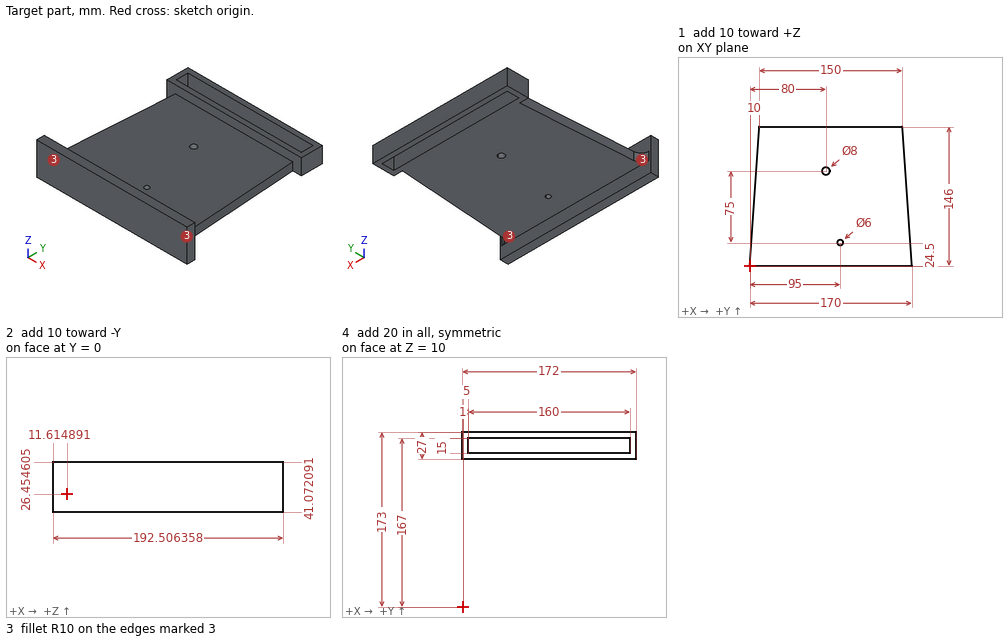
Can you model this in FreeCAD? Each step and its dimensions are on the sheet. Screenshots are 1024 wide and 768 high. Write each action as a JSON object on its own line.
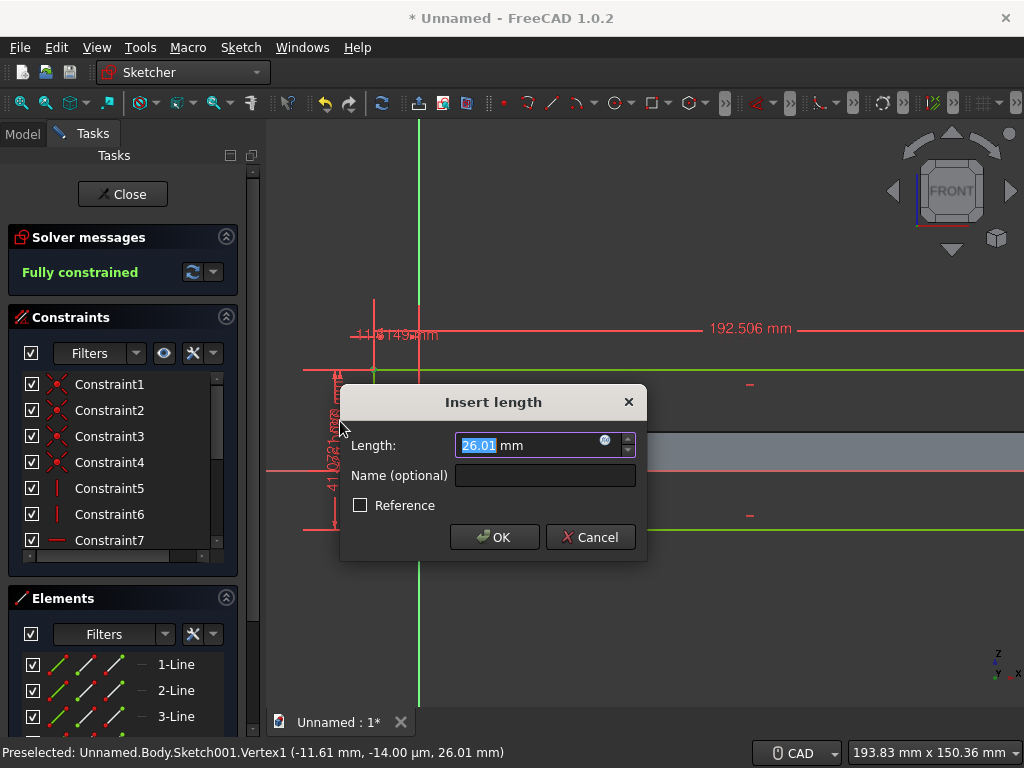
{"action": "type", "text": "26.454605"}
{"action": "key", "text": "Return"}
{"action": "key", "text": "Escape"}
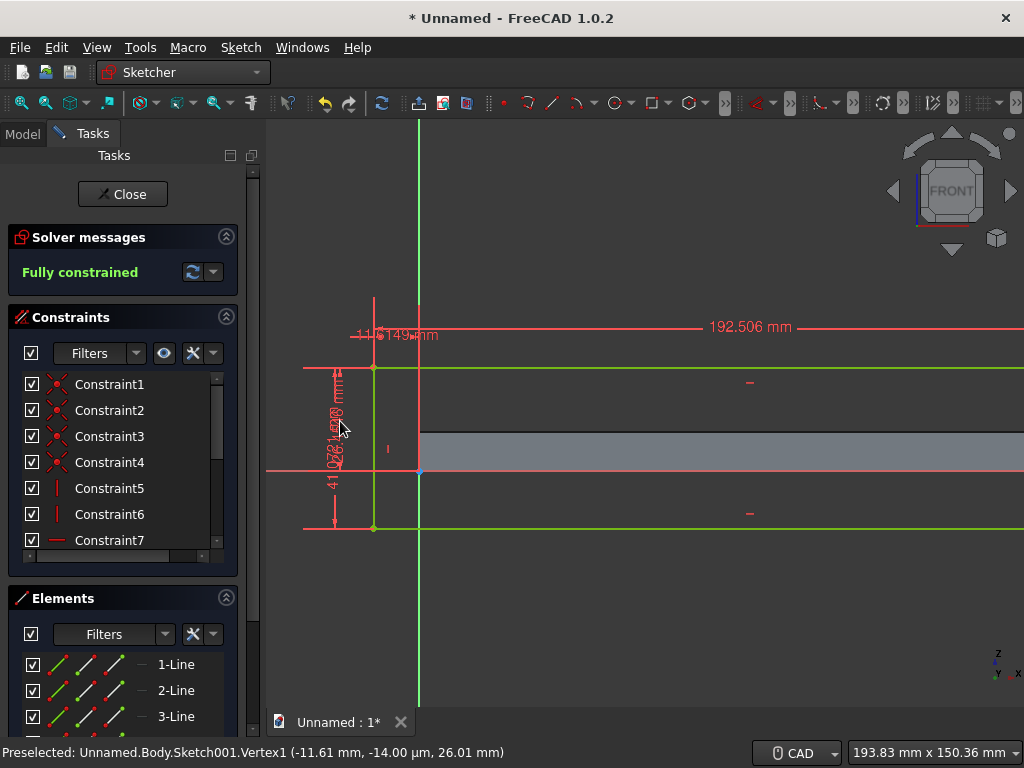
{"action": "left_click", "coordinate": [123, 194]}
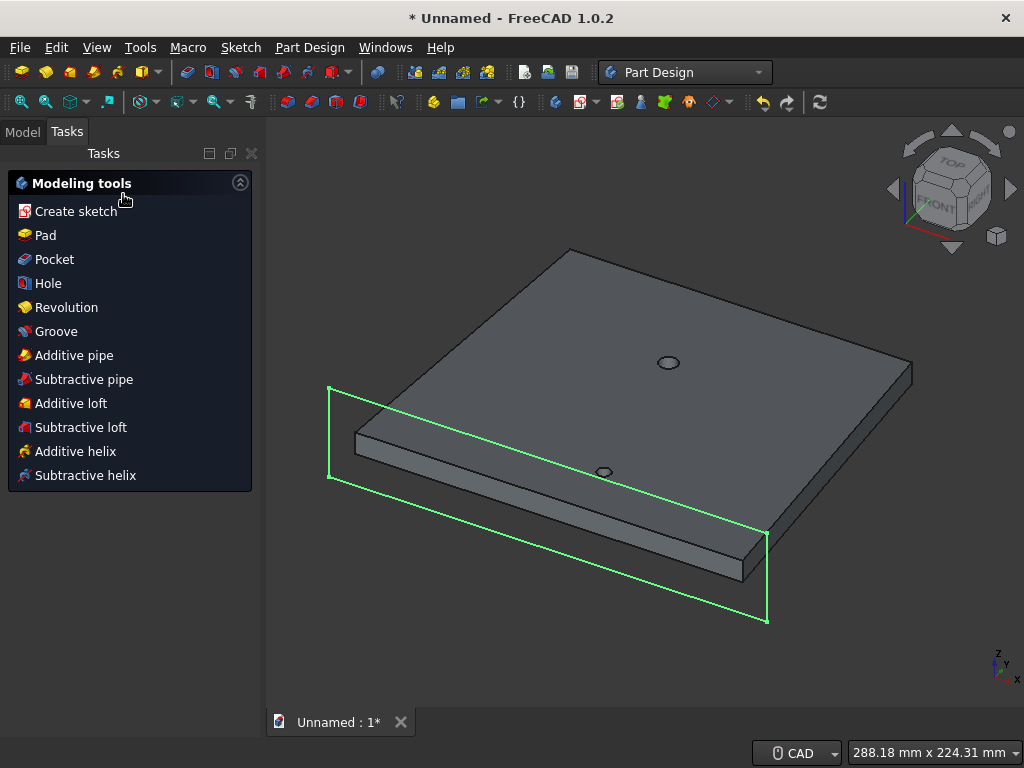
{"action": "left_click", "coordinate": [22, 72]}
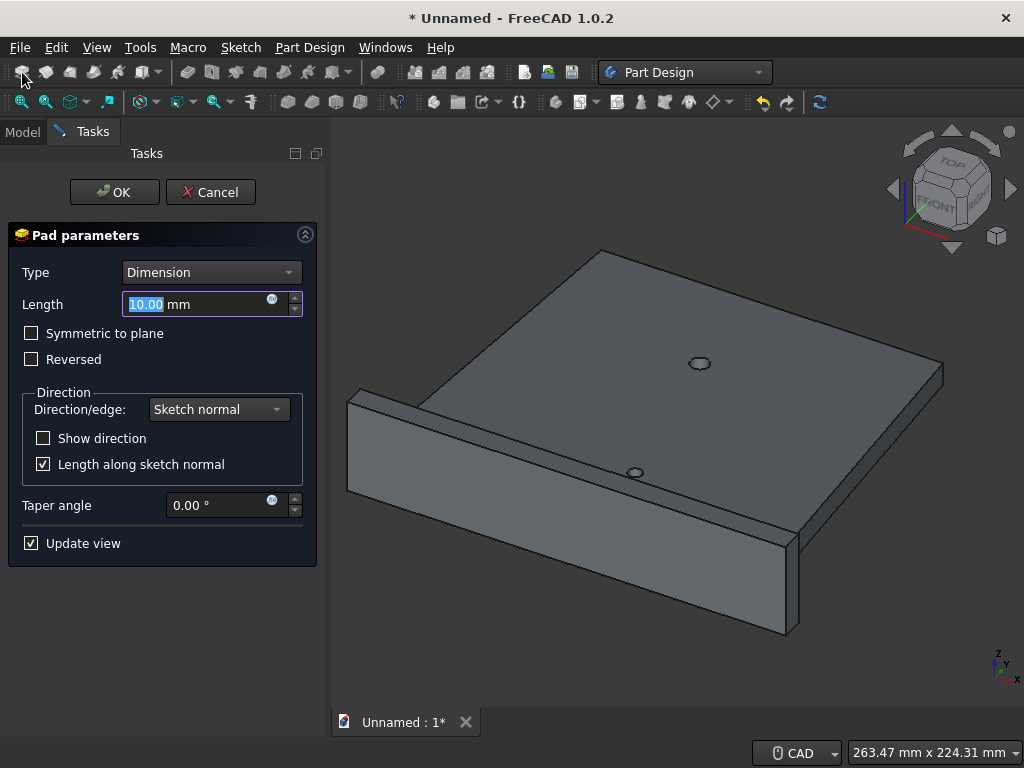
{"action": "type", "text": "10"}
{"action": "key", "text": "Tab"}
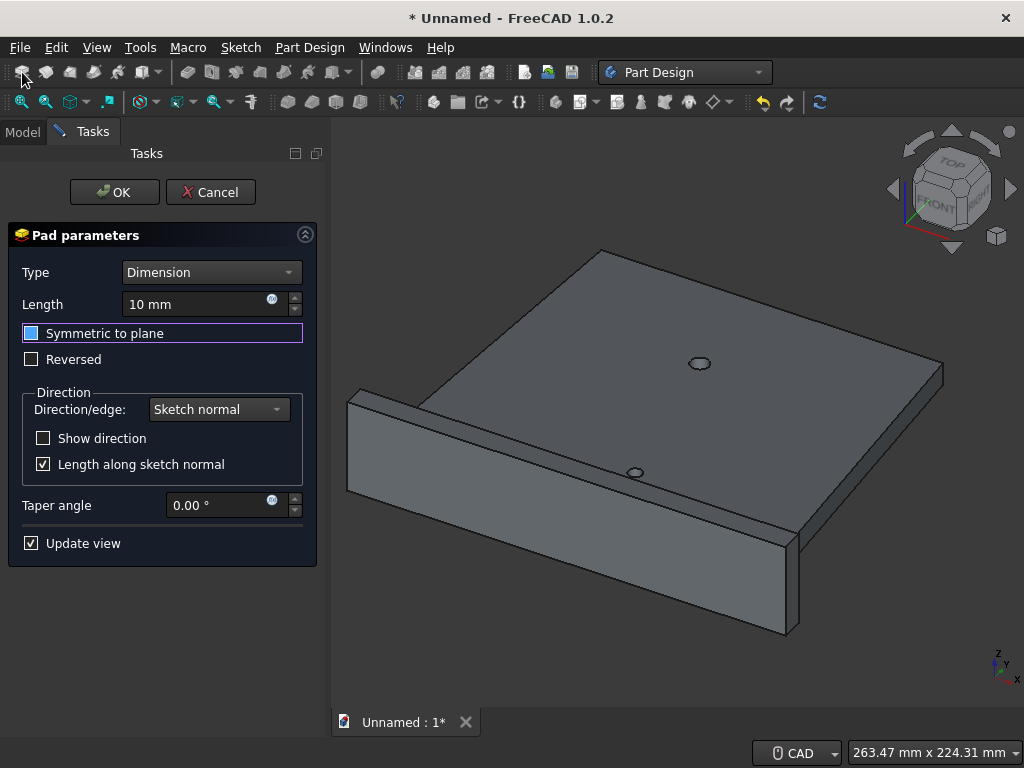
{"action": "left_click", "coordinate": [115, 192]}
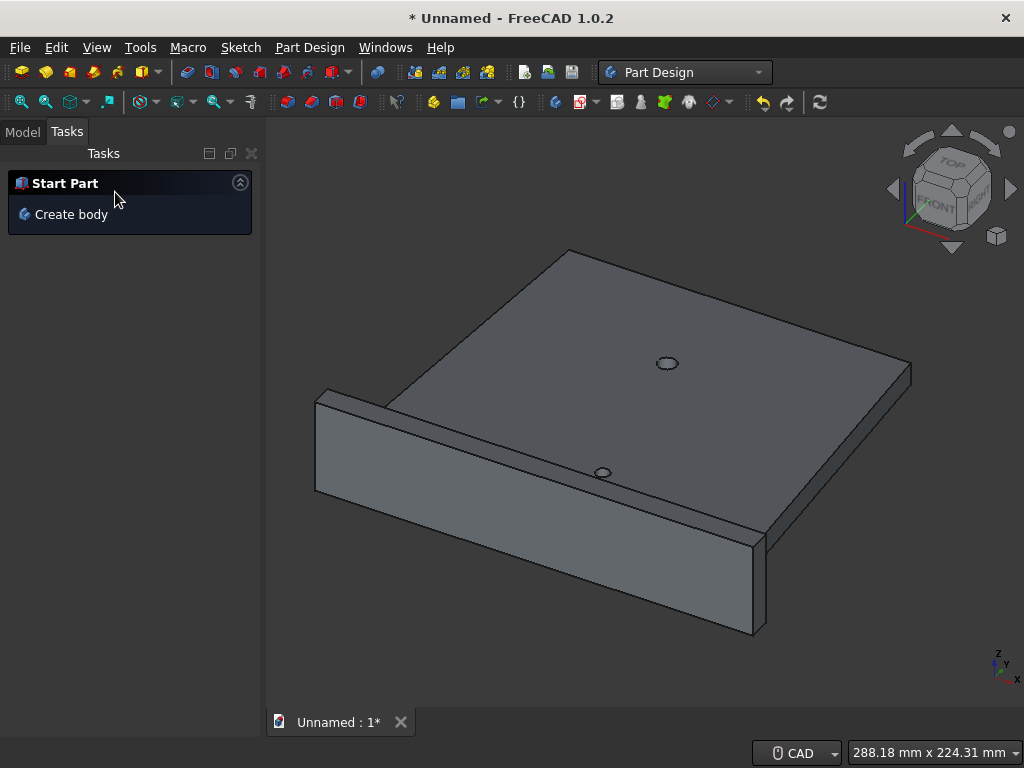
{"action": "key", "text": "0"}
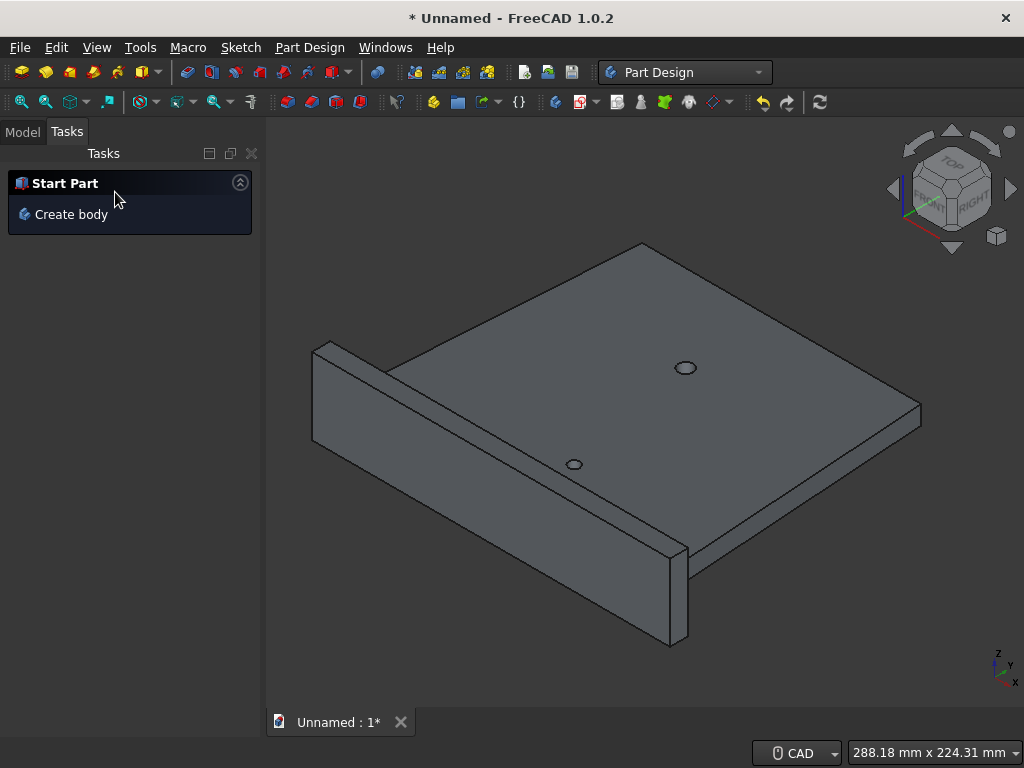
{"action": "key", "text": "2"}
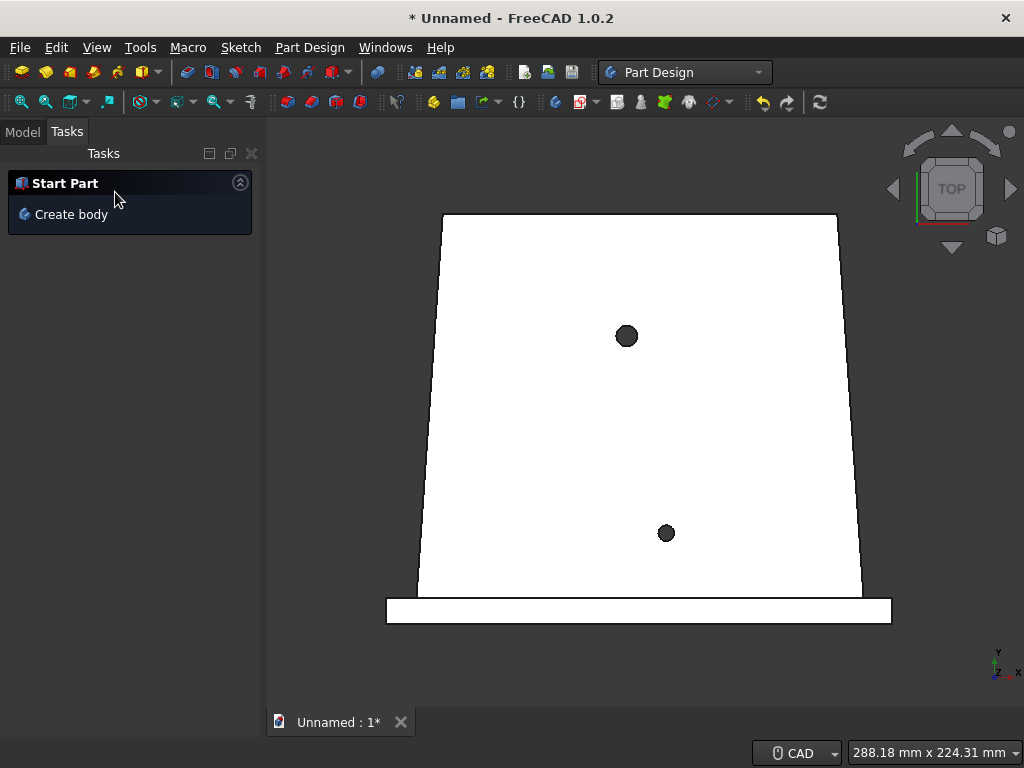
{"action": "key", "text": "1"}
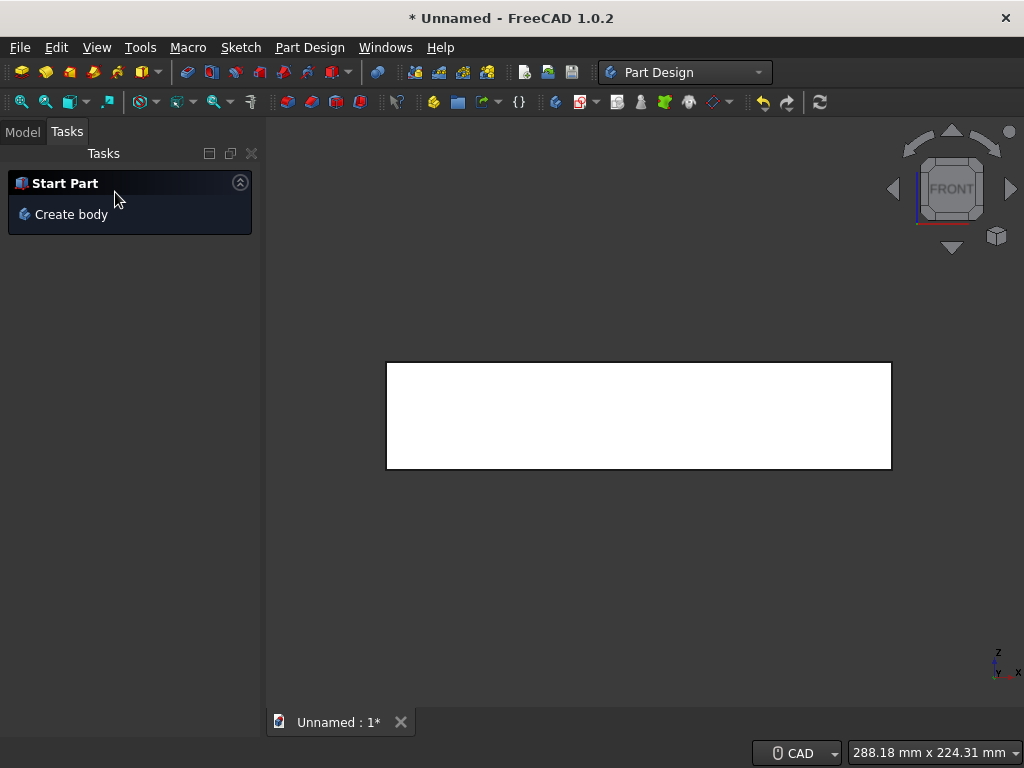
{"action": "key", "text": "3"}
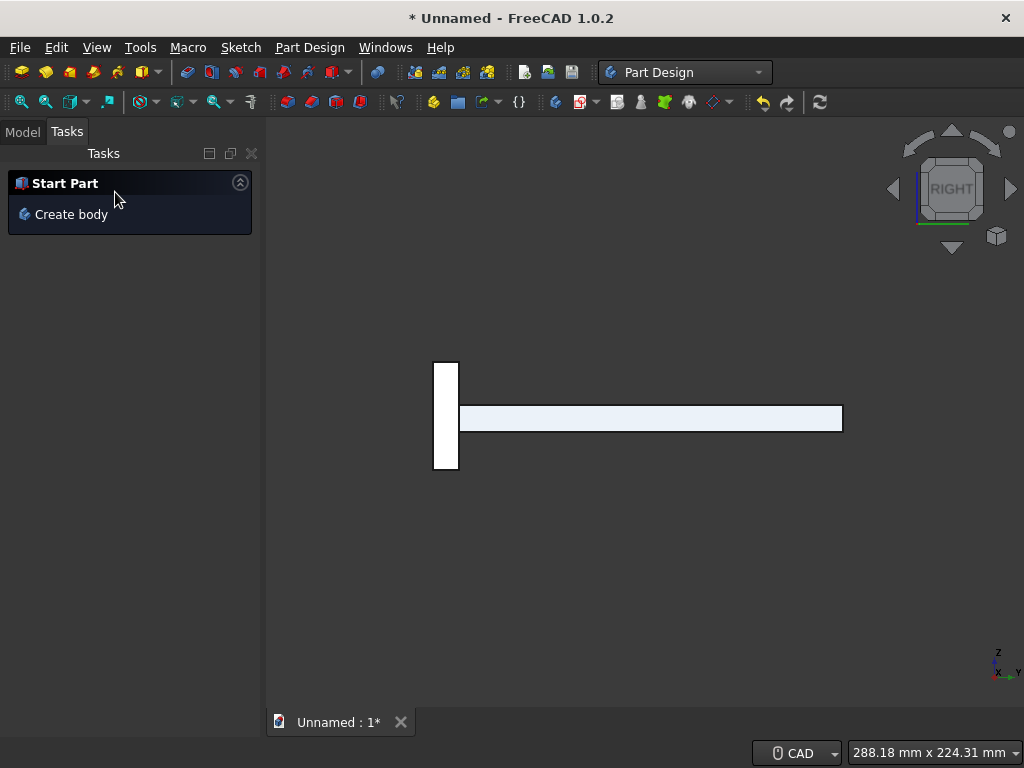
{"action": "key", "text": "5"}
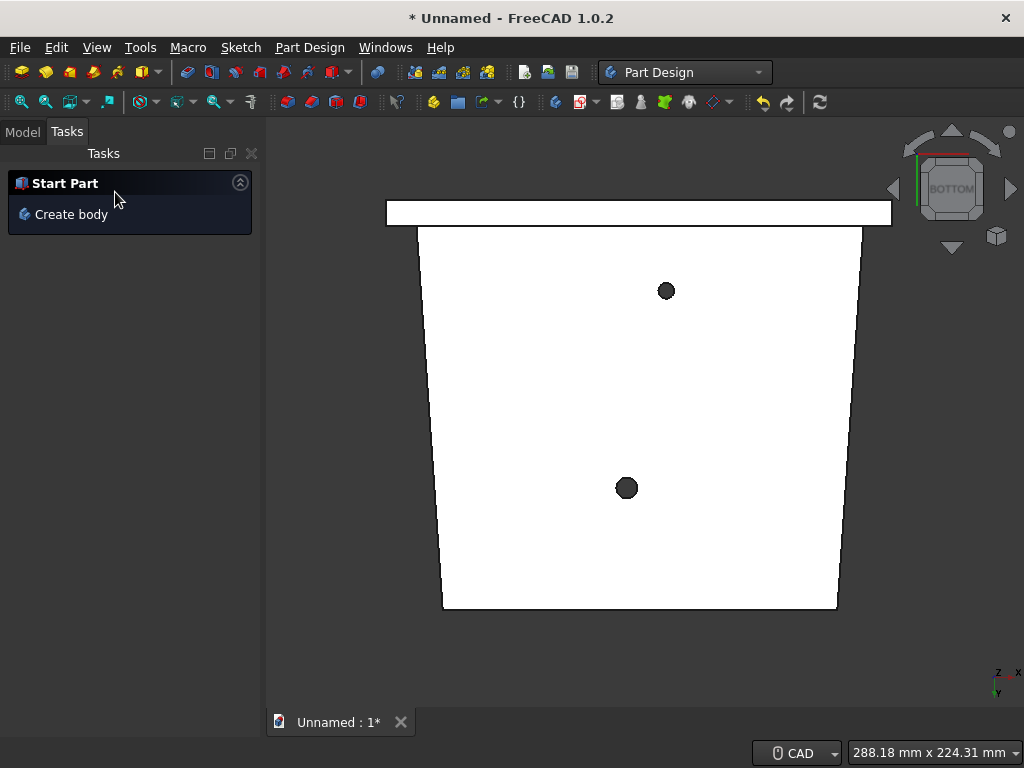
{"action": "key", "text": "4"}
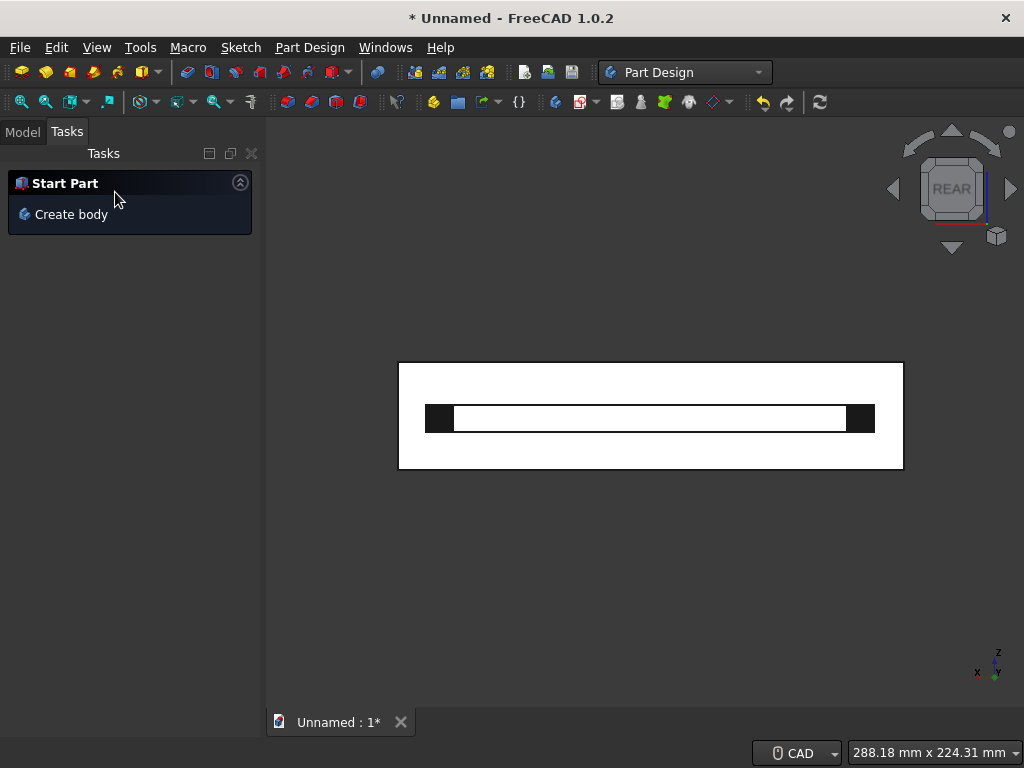
{"action": "key", "text": "6"}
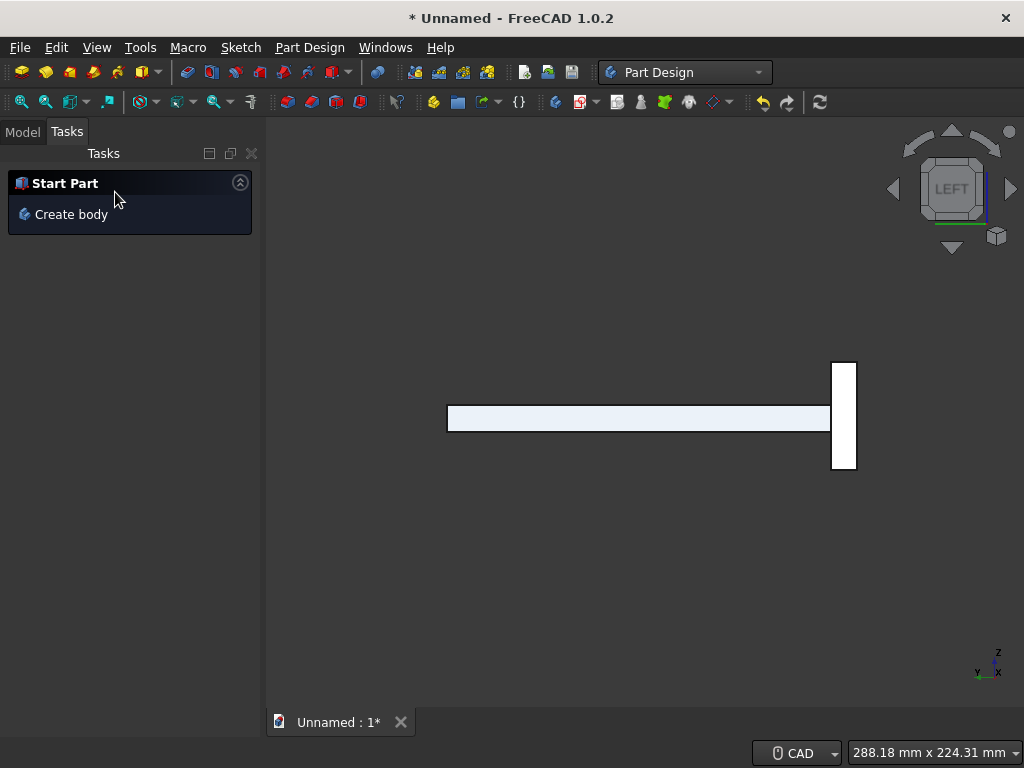
{"action": "key", "text": "v 3"}